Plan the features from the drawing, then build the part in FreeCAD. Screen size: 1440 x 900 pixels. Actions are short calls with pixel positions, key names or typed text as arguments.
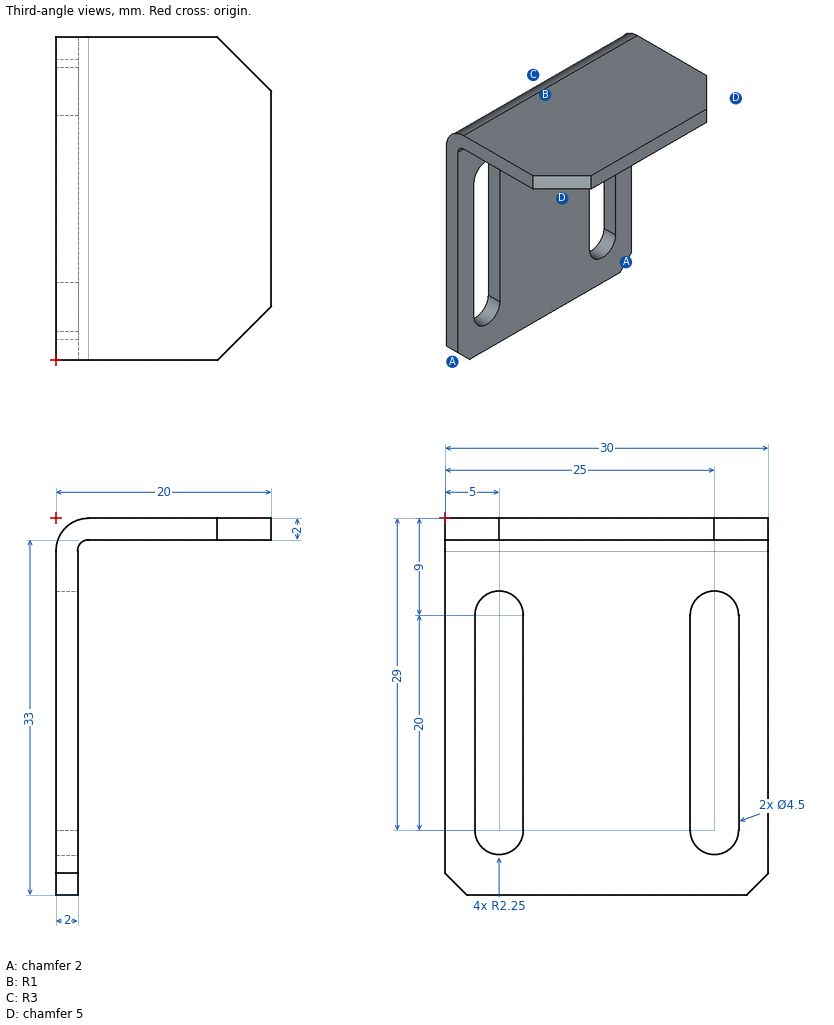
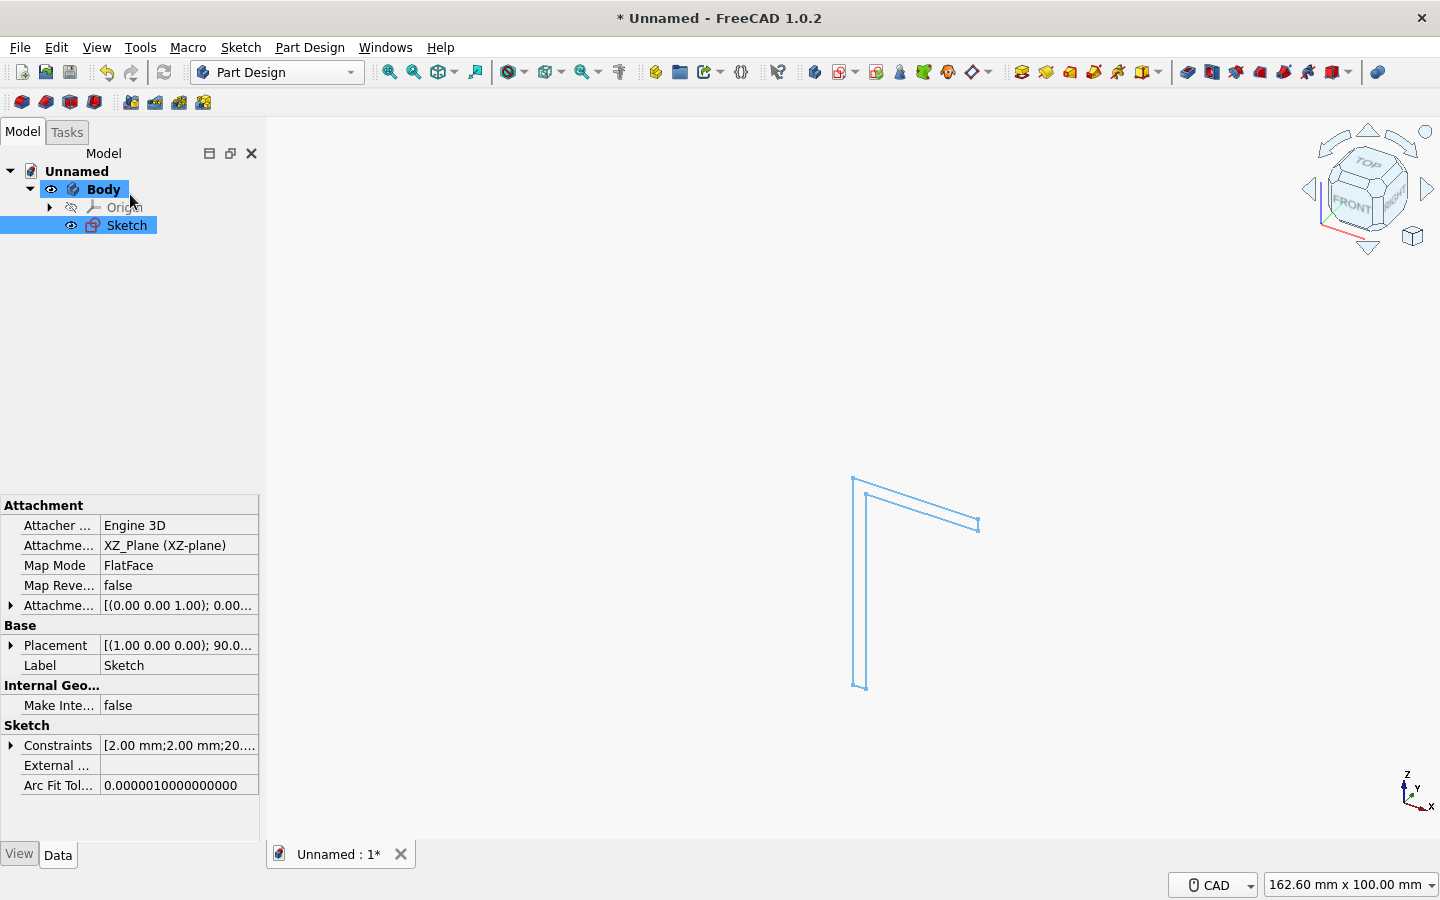
click(1022, 72)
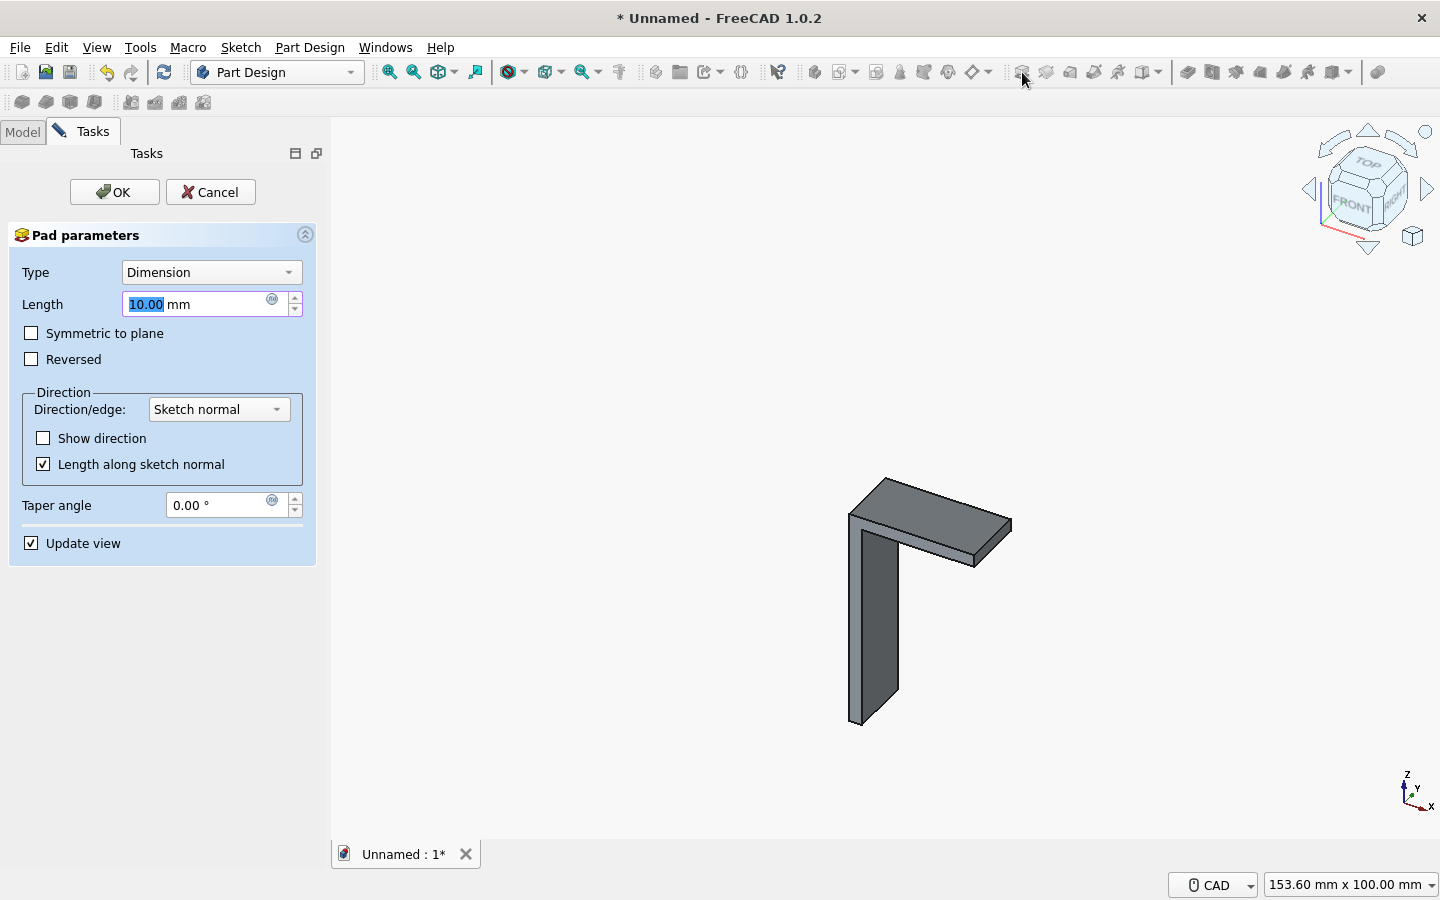
text(30)
key(Tab)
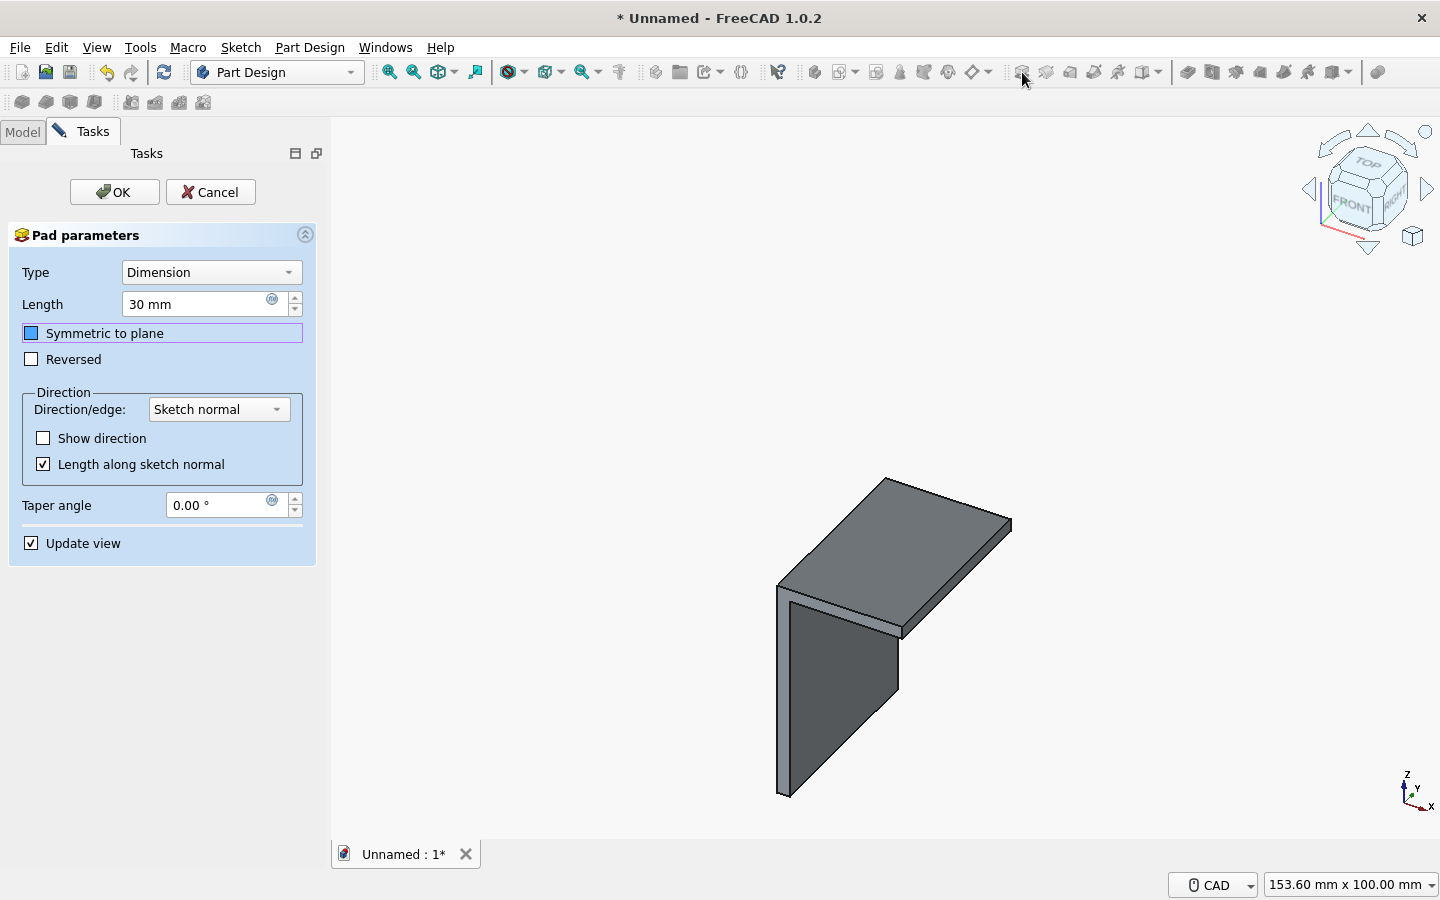
click(30, 359)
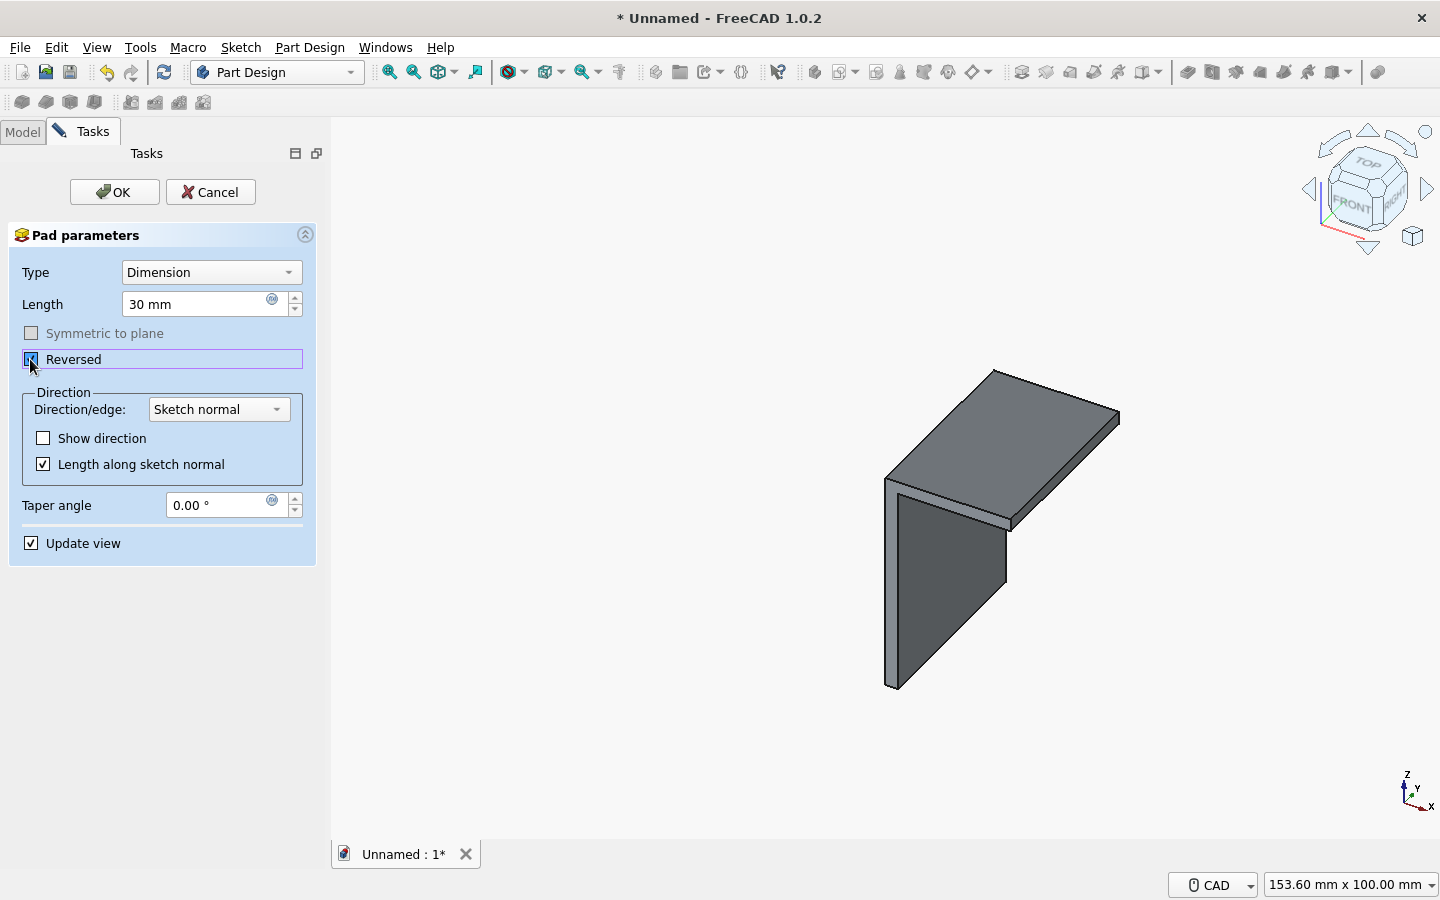
click(115, 192)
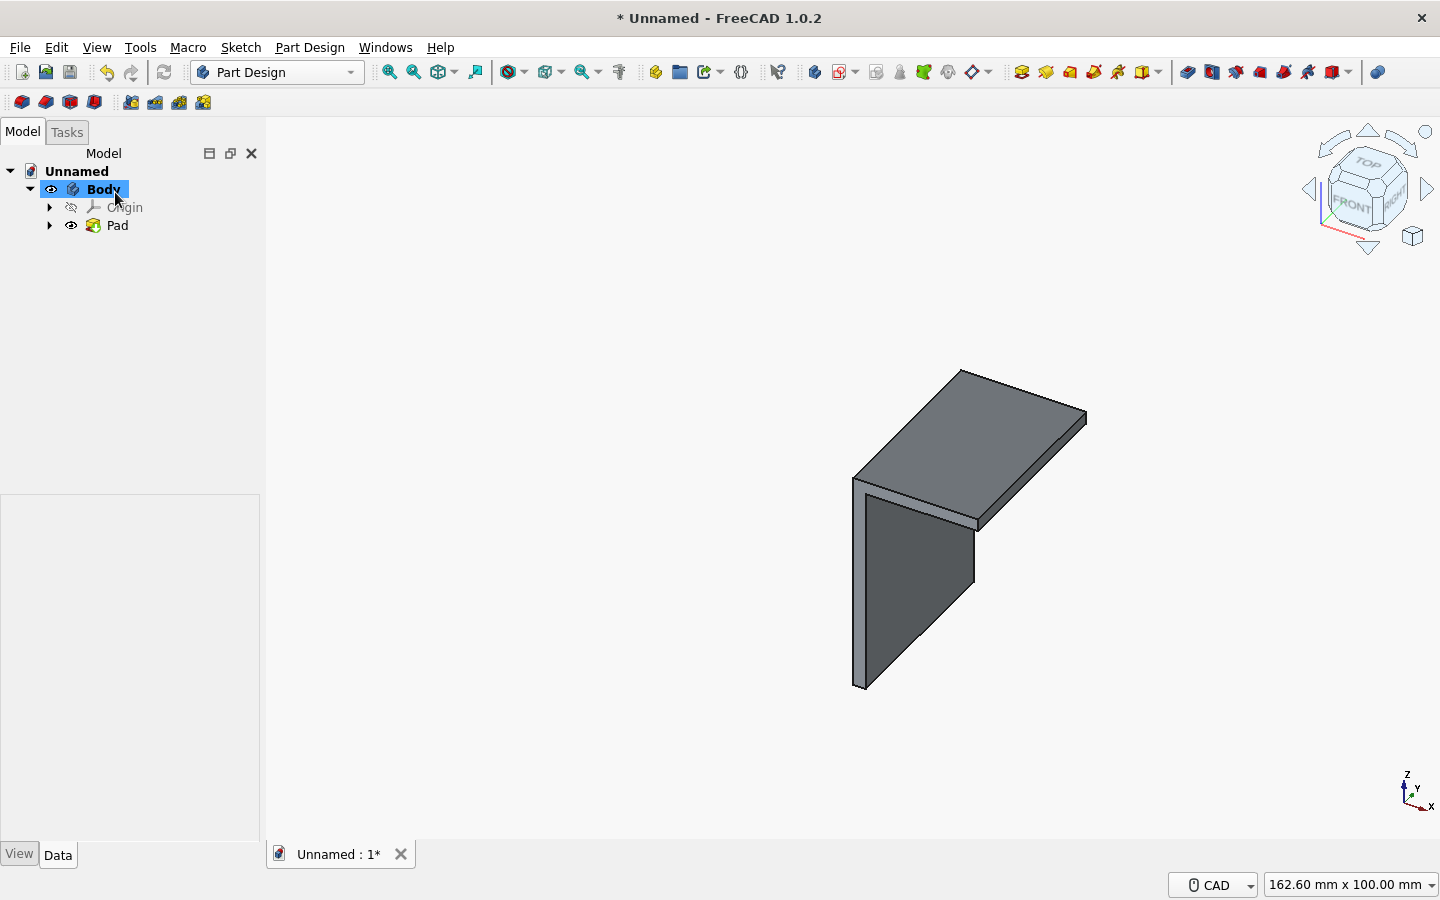
click(920, 537)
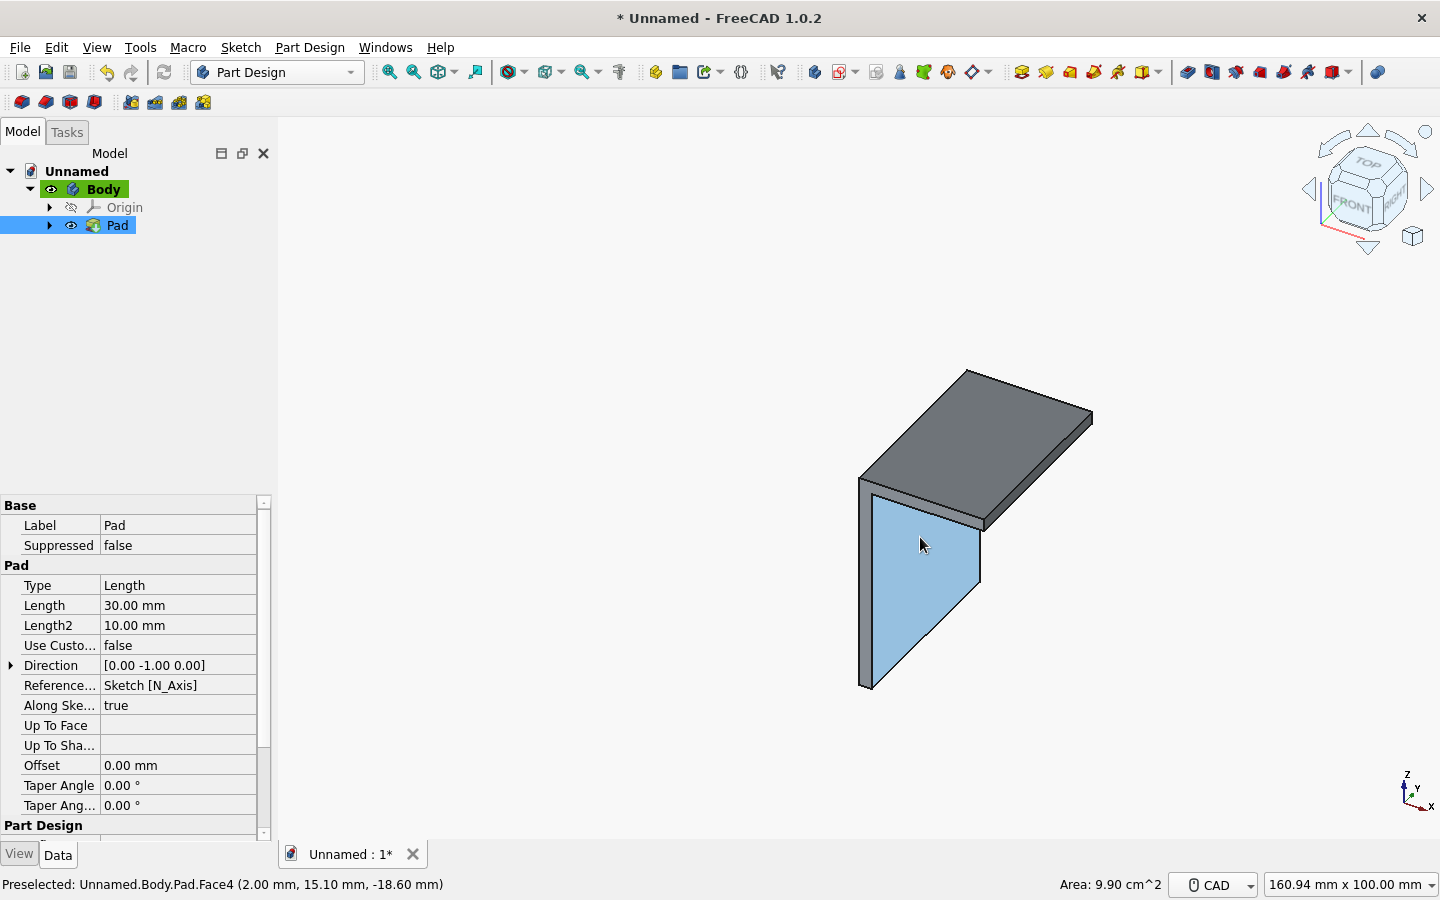
click(840, 72)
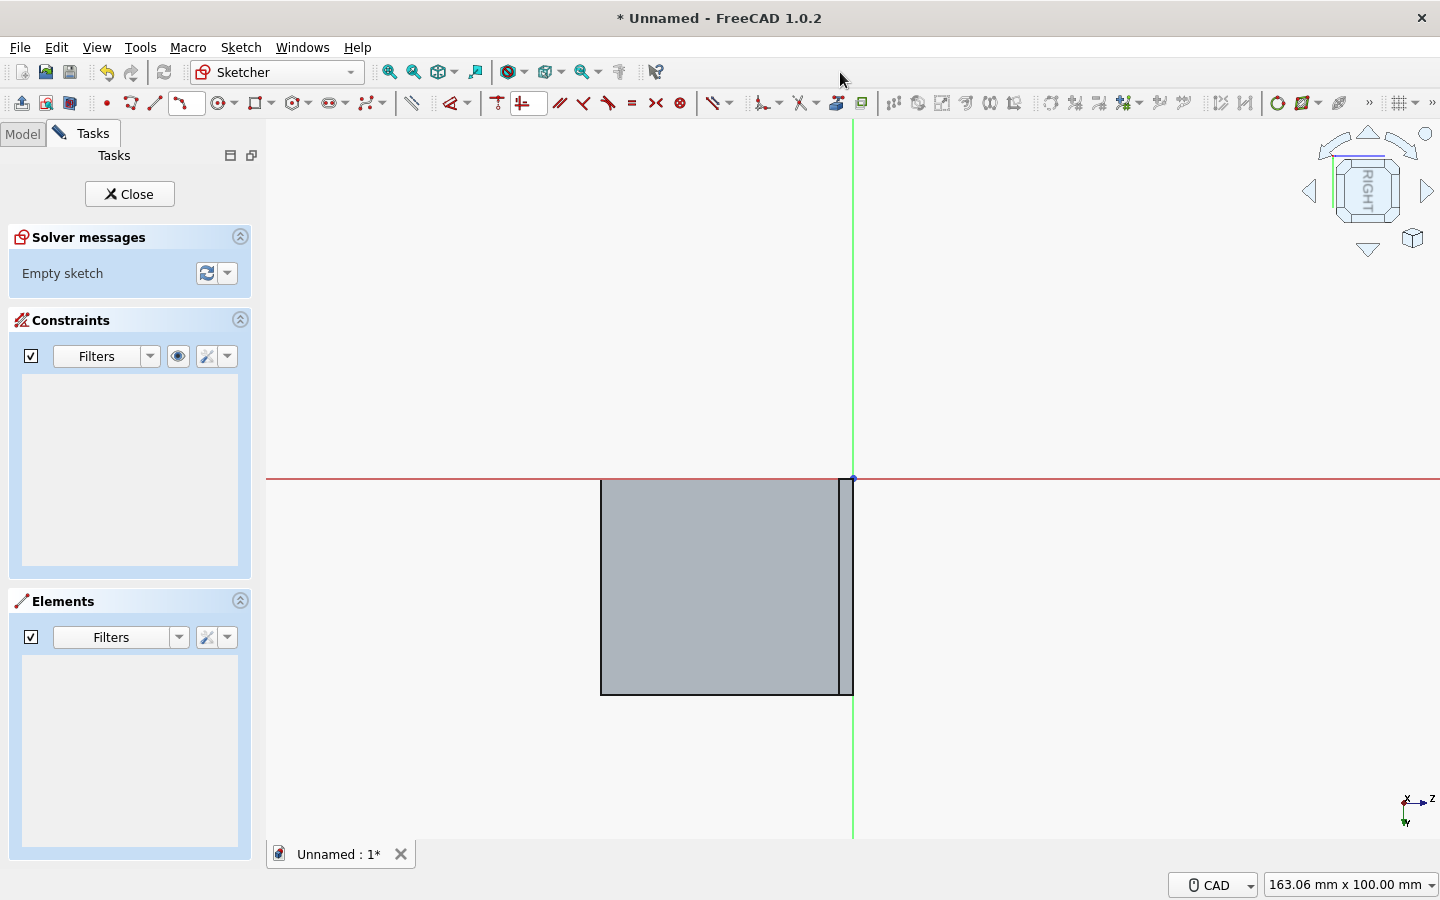
click(70, 104)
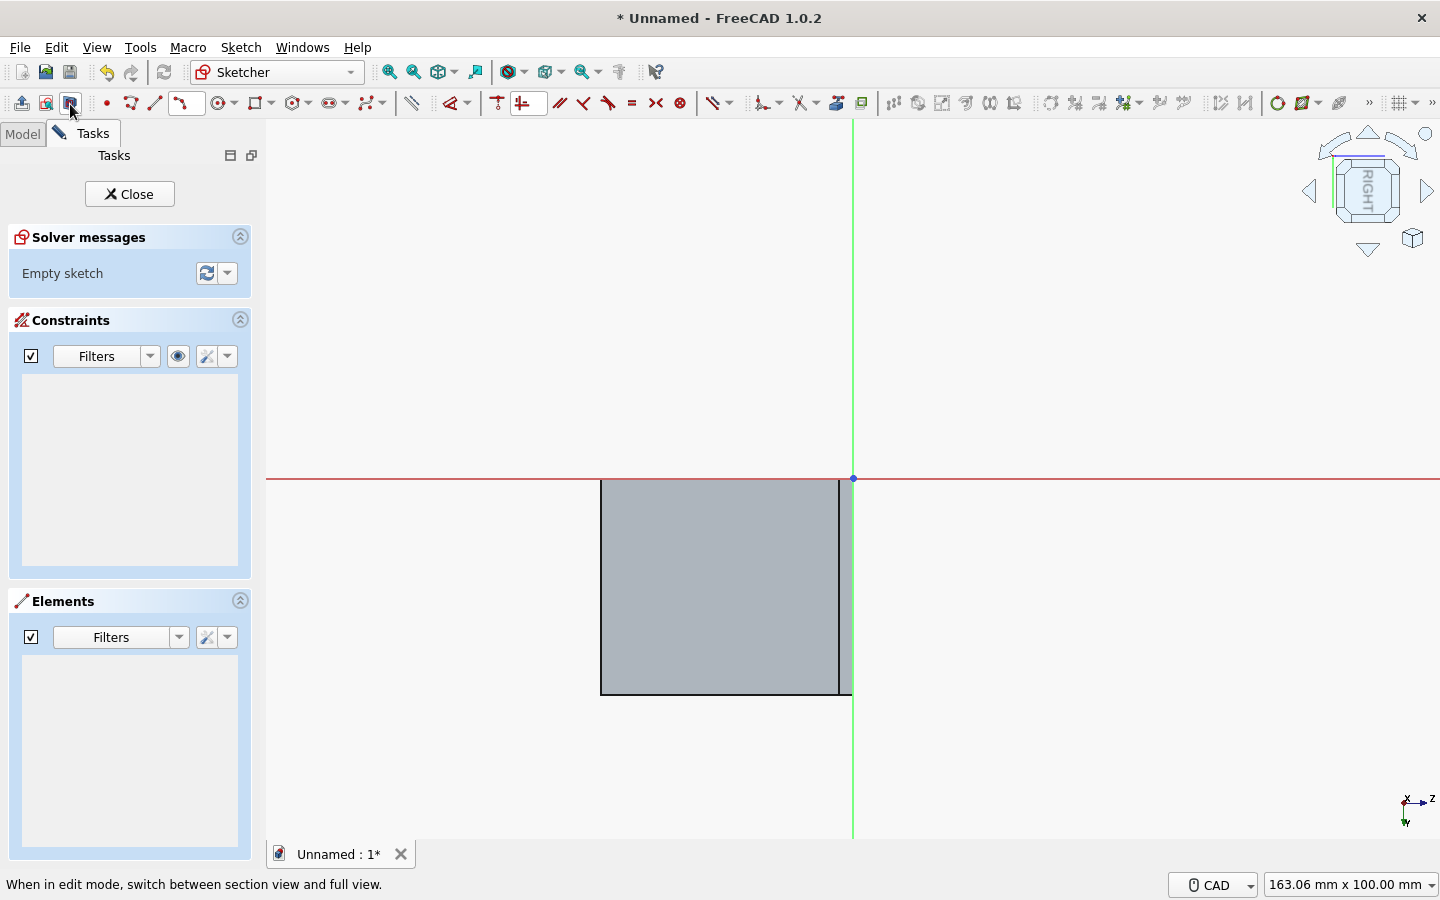
scroll(705, 657, up, 4)